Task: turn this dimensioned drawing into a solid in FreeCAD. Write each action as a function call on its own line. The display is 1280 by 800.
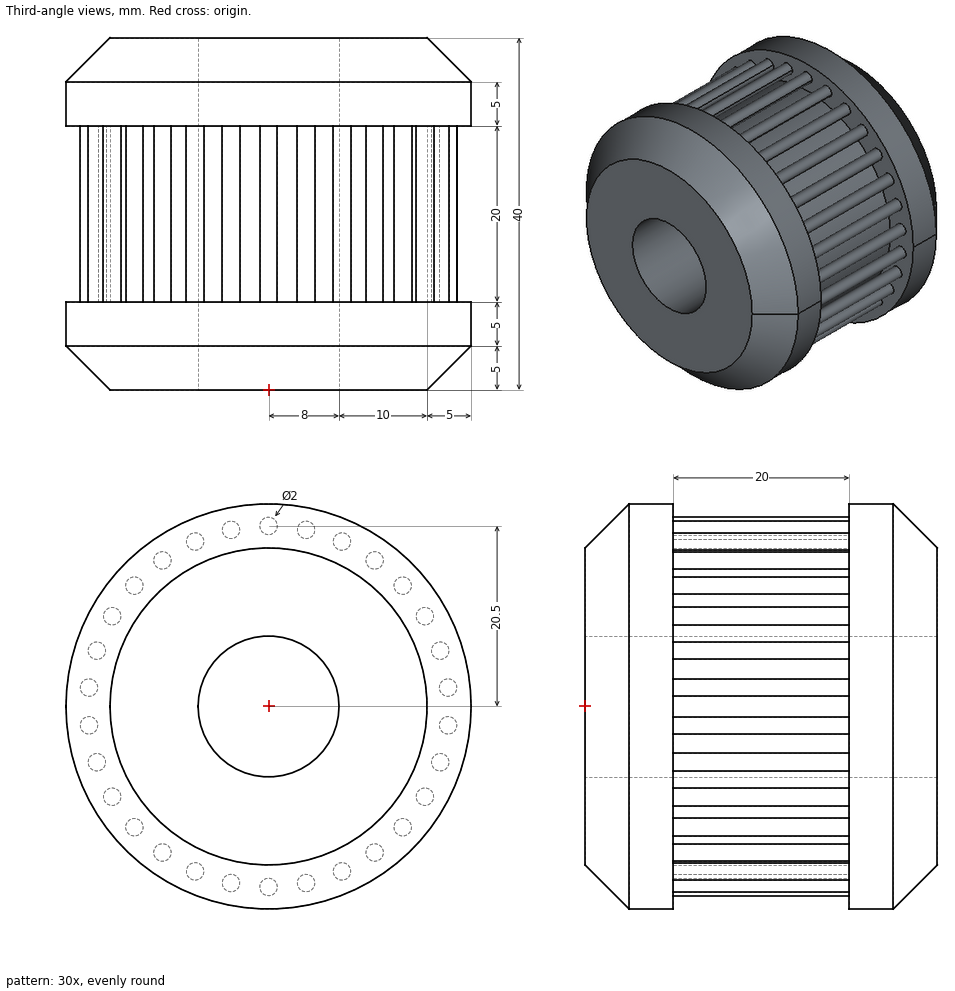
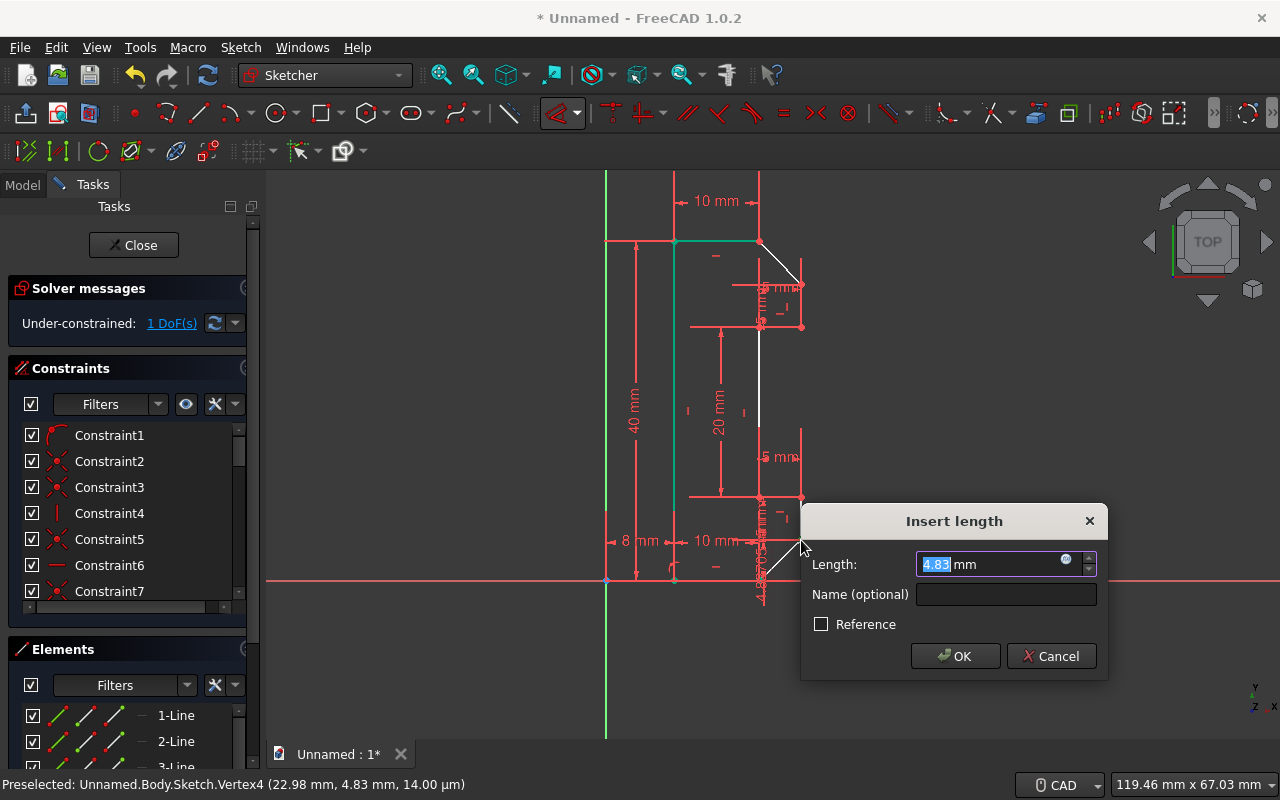
text(5)
key(Return)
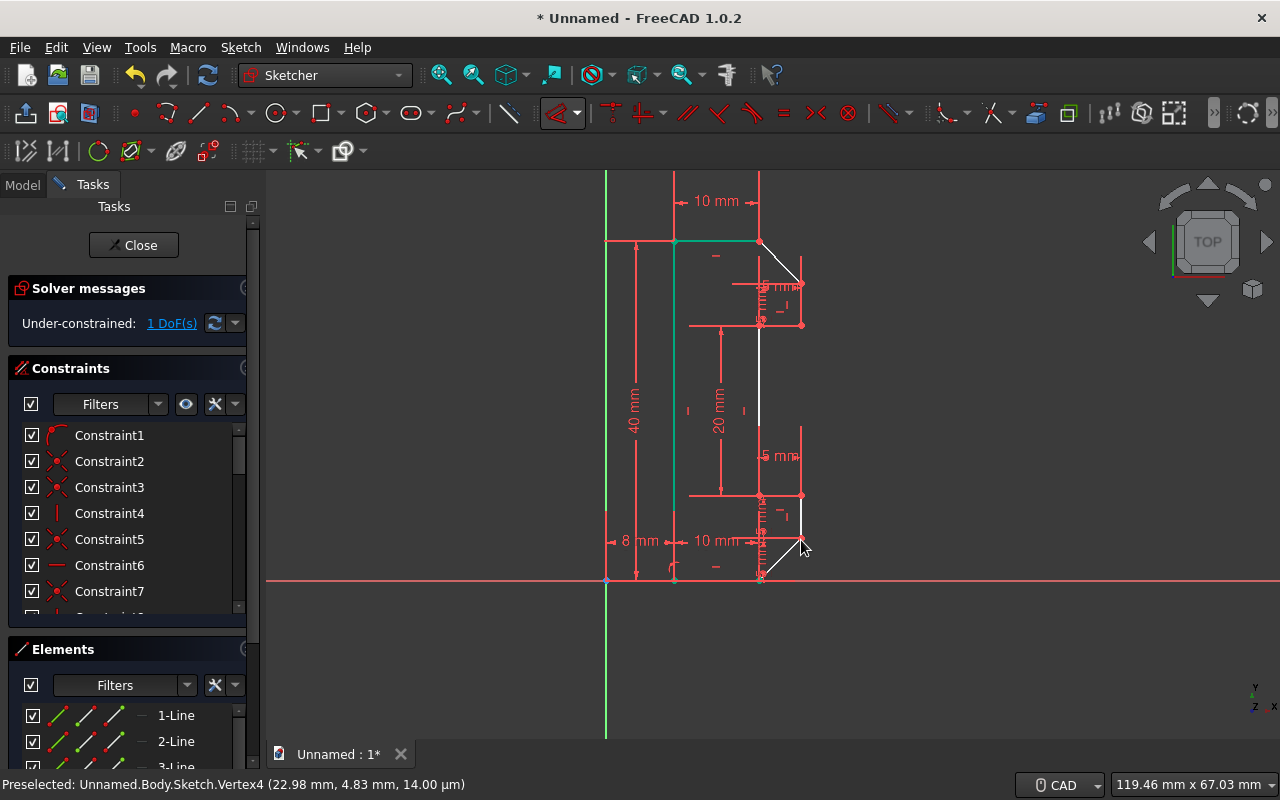
click(772, 568)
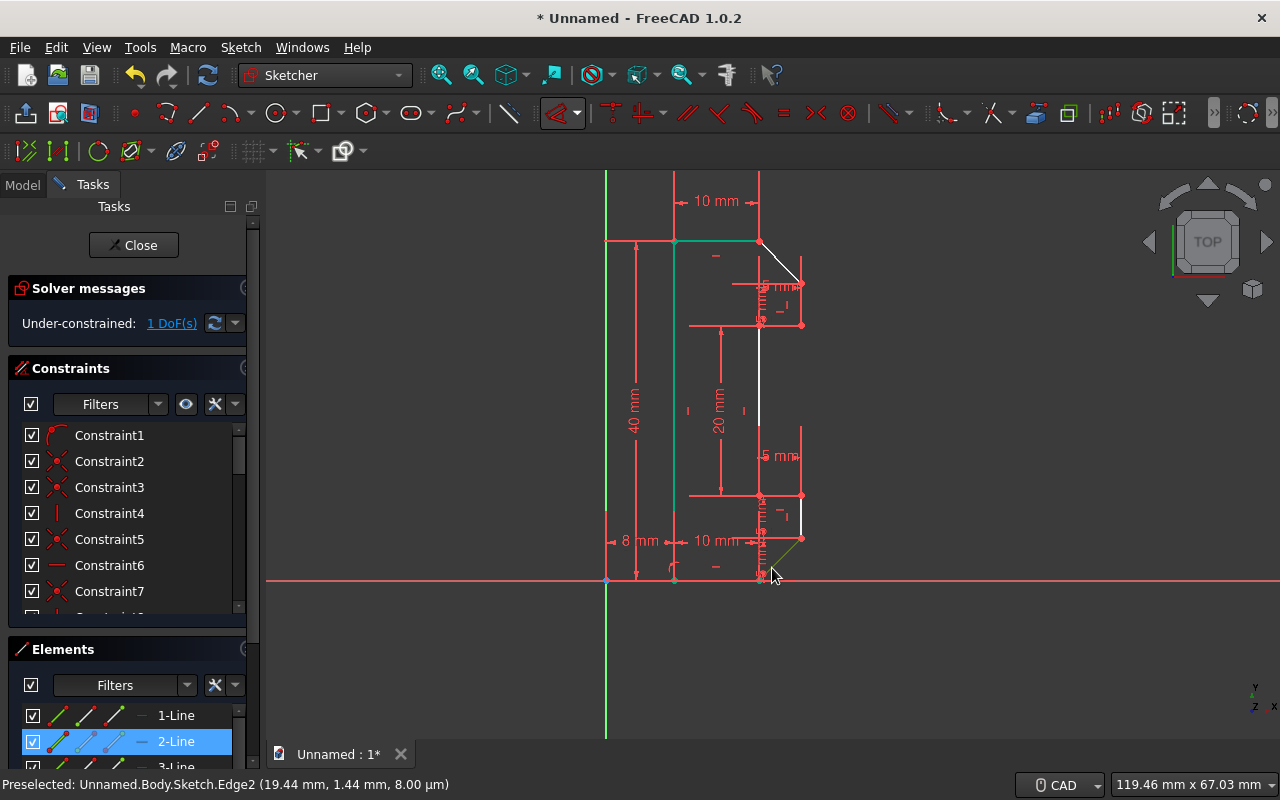
key(l)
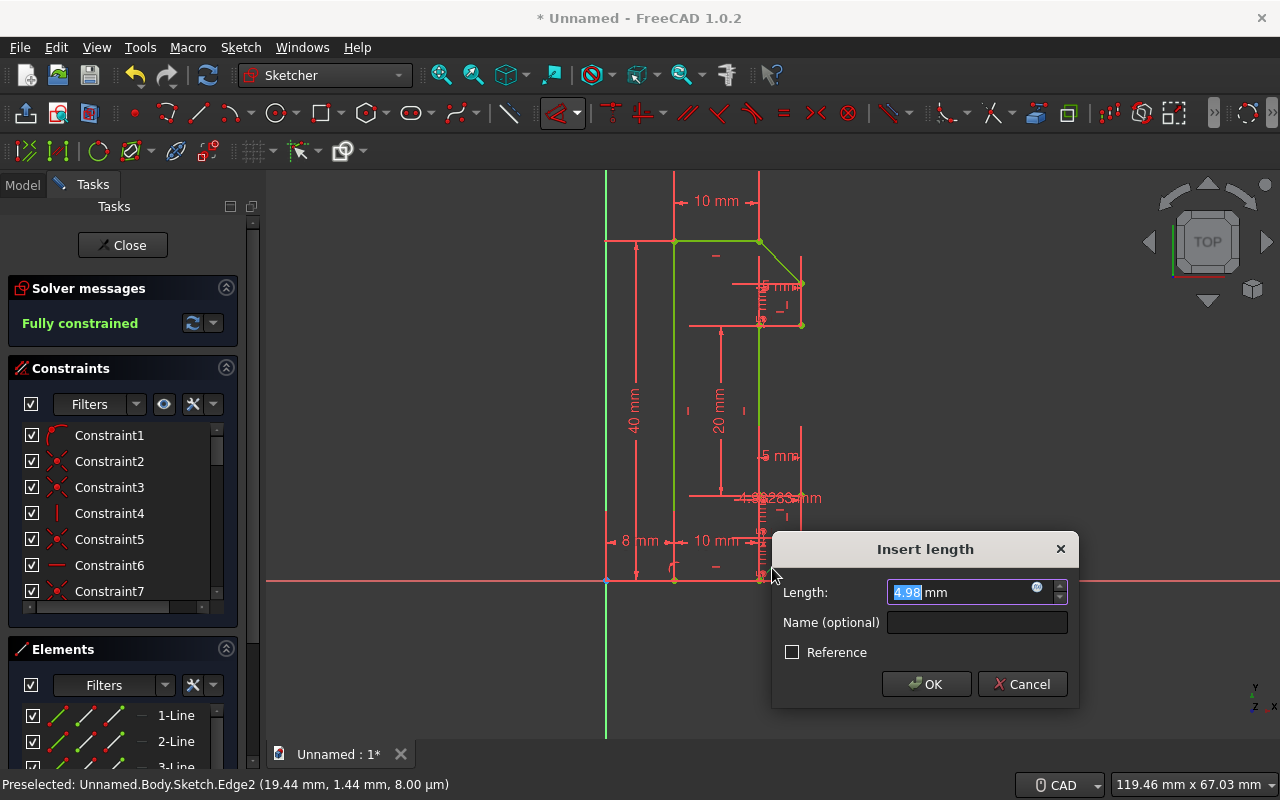
text(5)
key(Return)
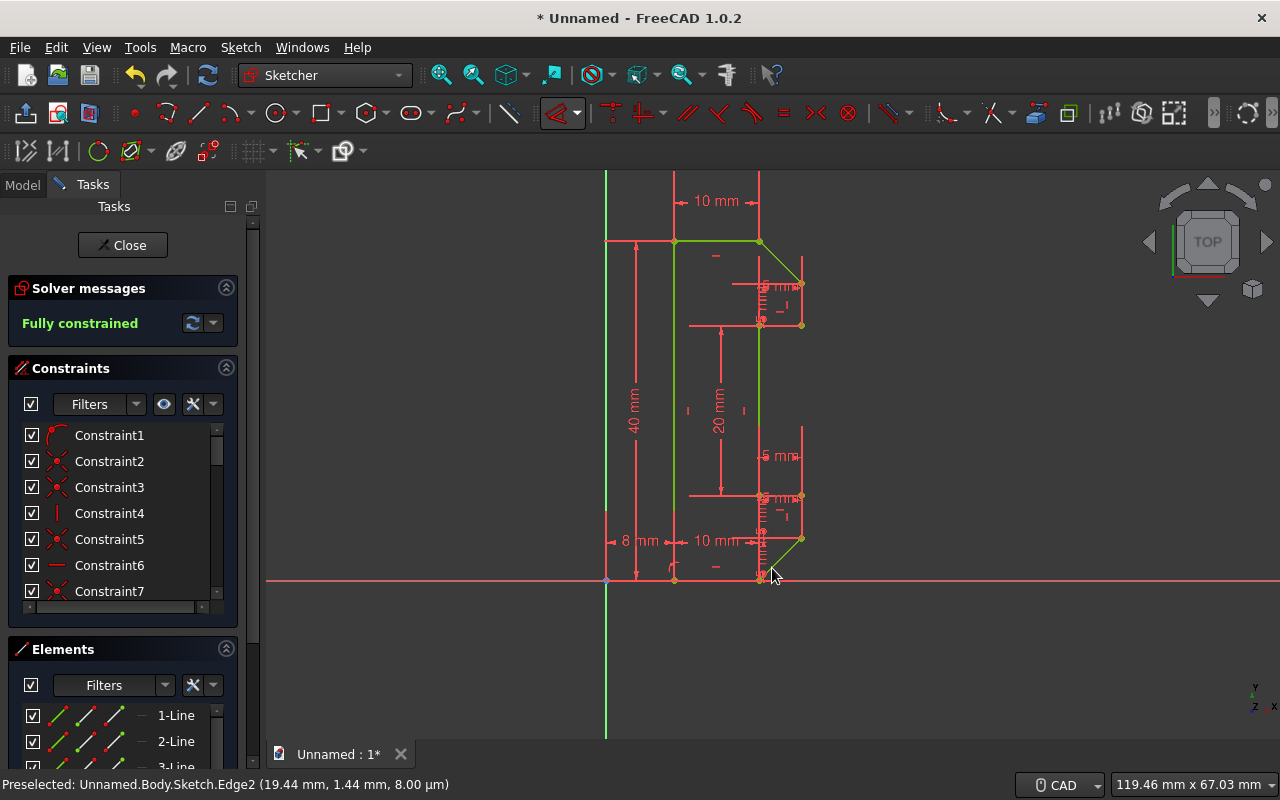
click(123, 245)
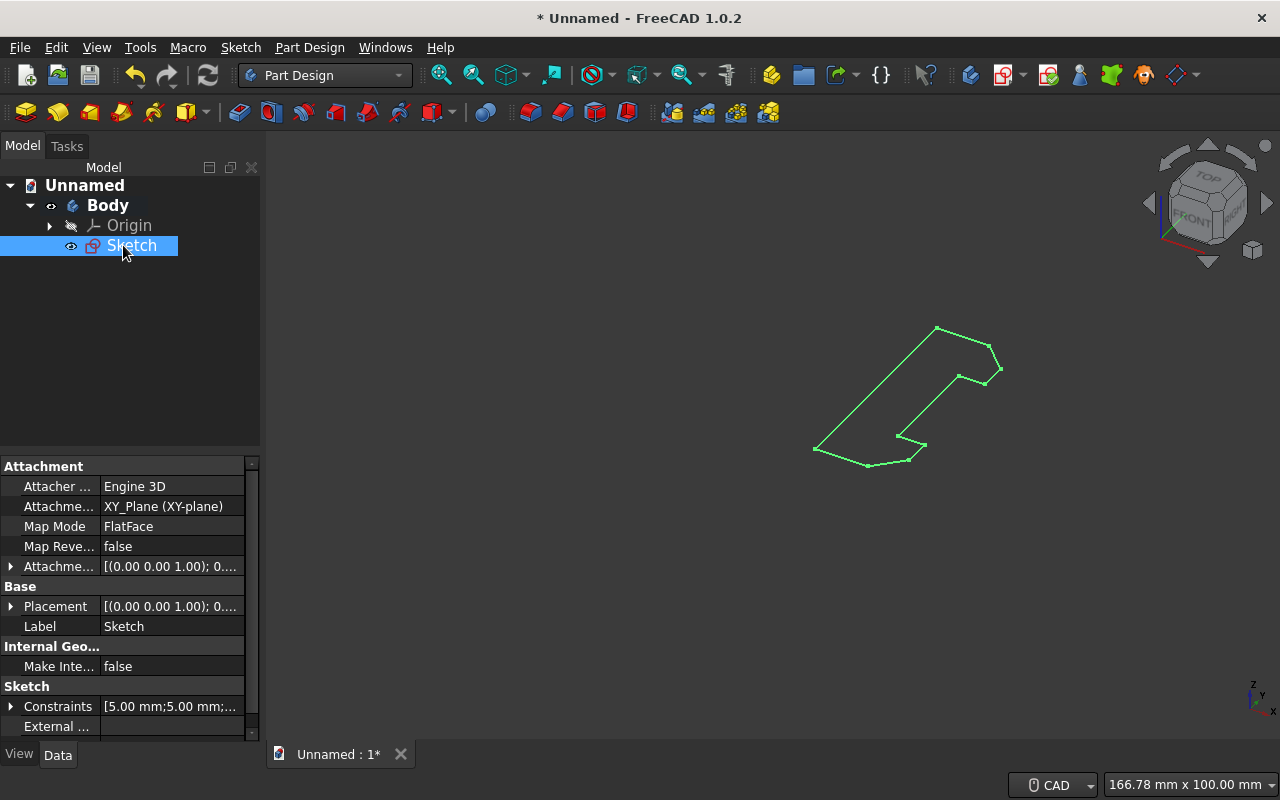
click(58, 112)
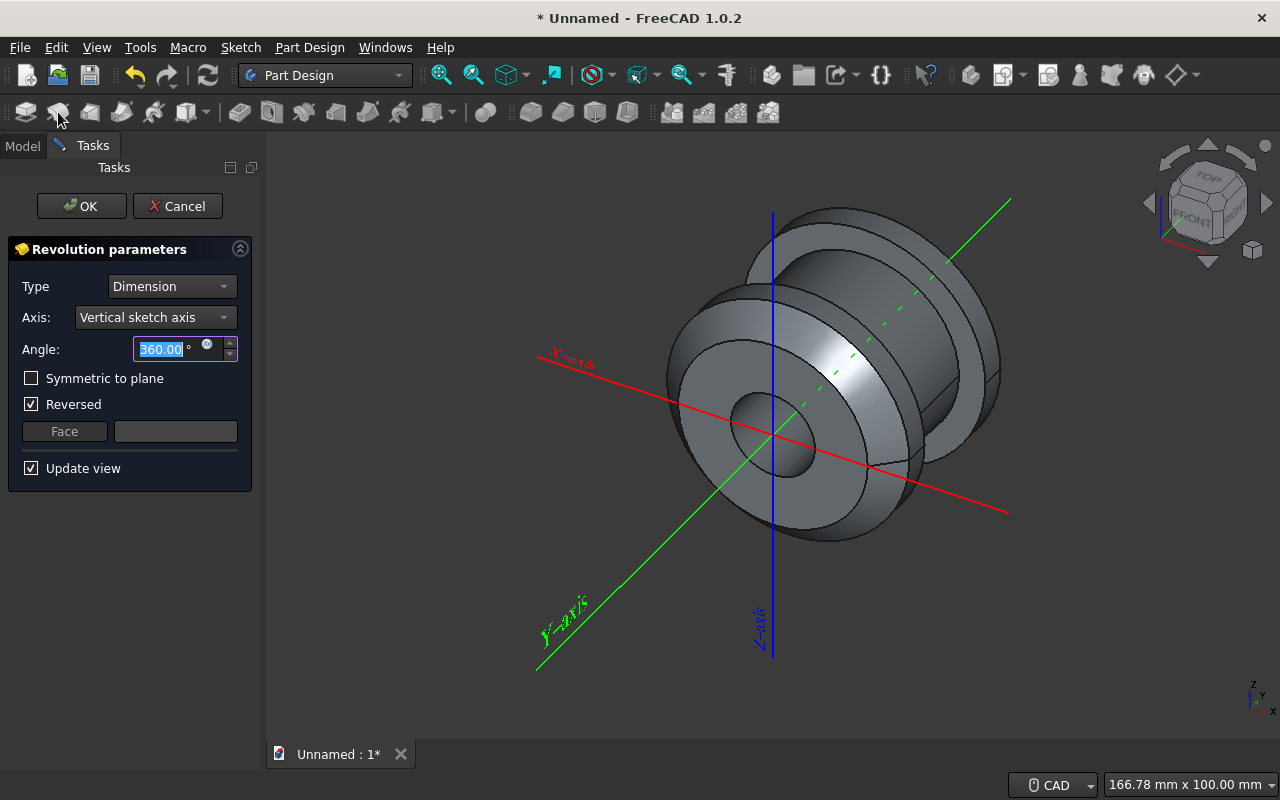
click(82, 206)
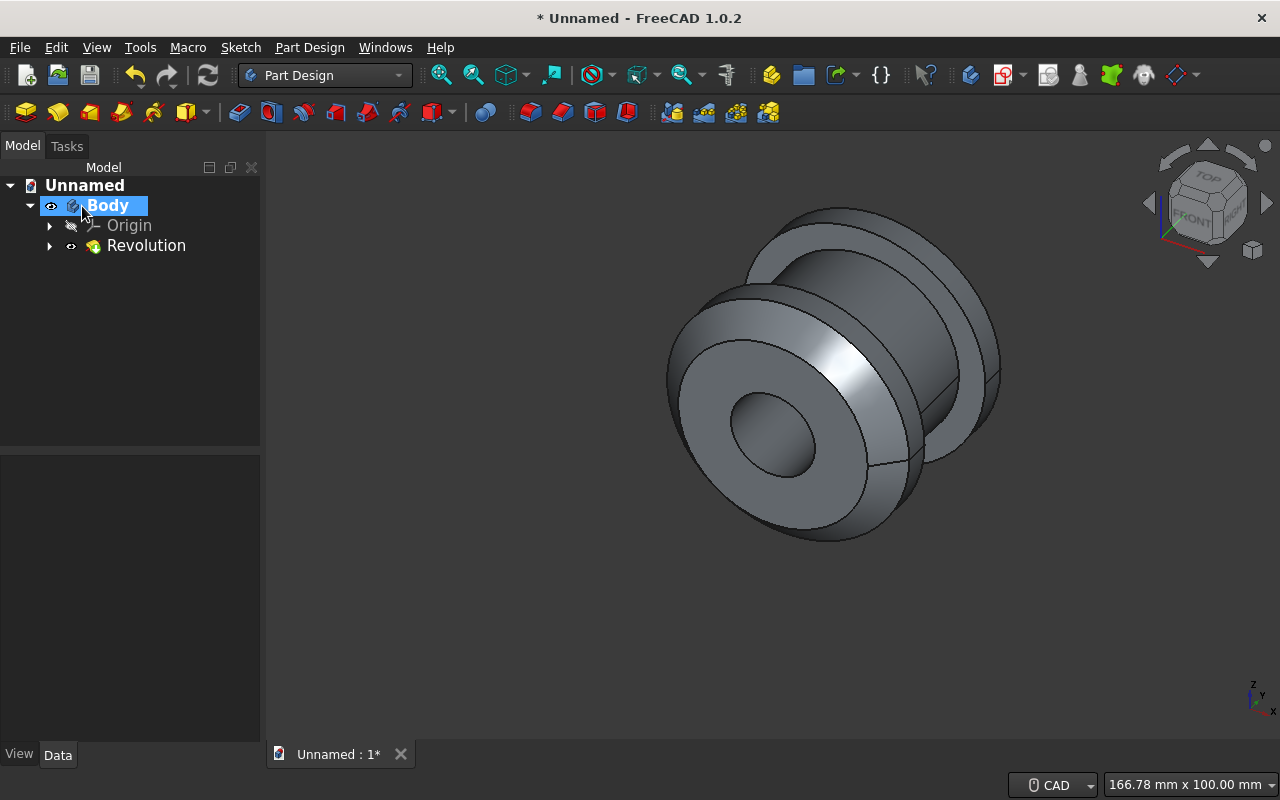
click(50, 226)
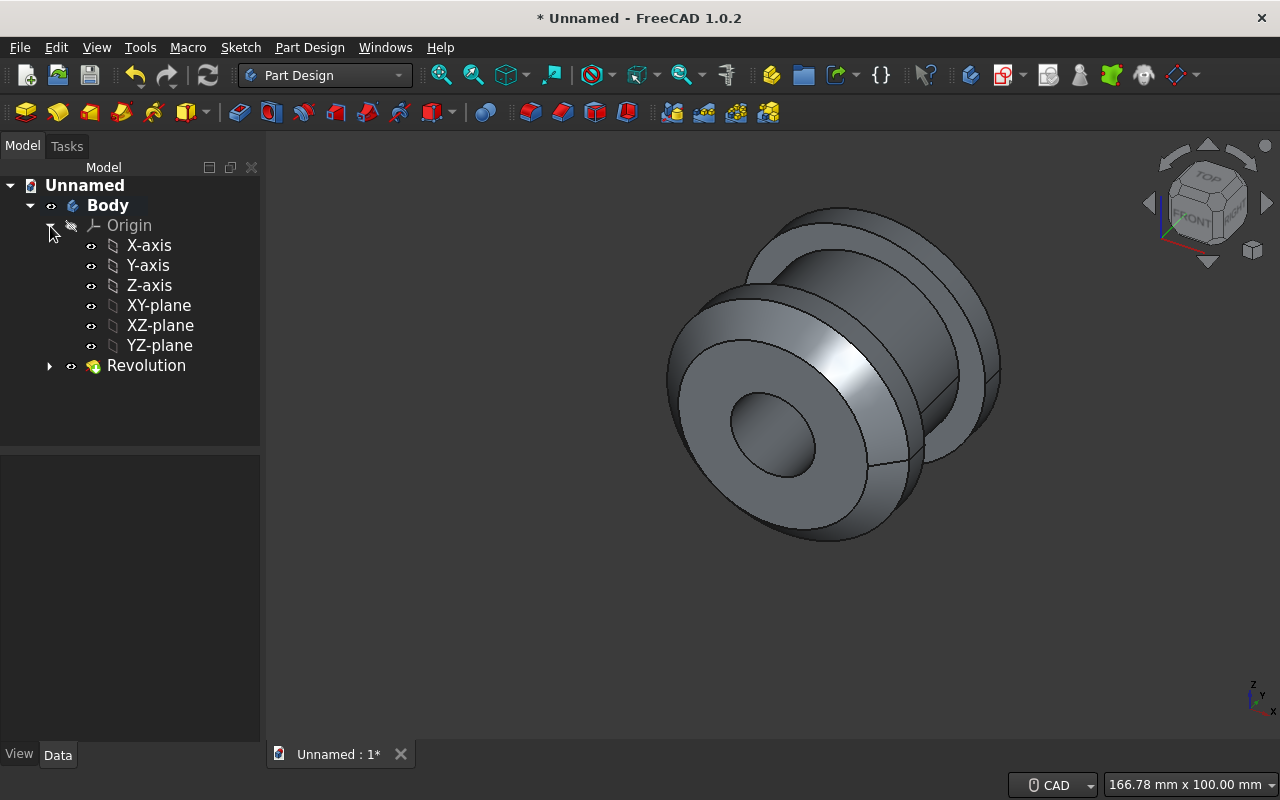
click(136, 326)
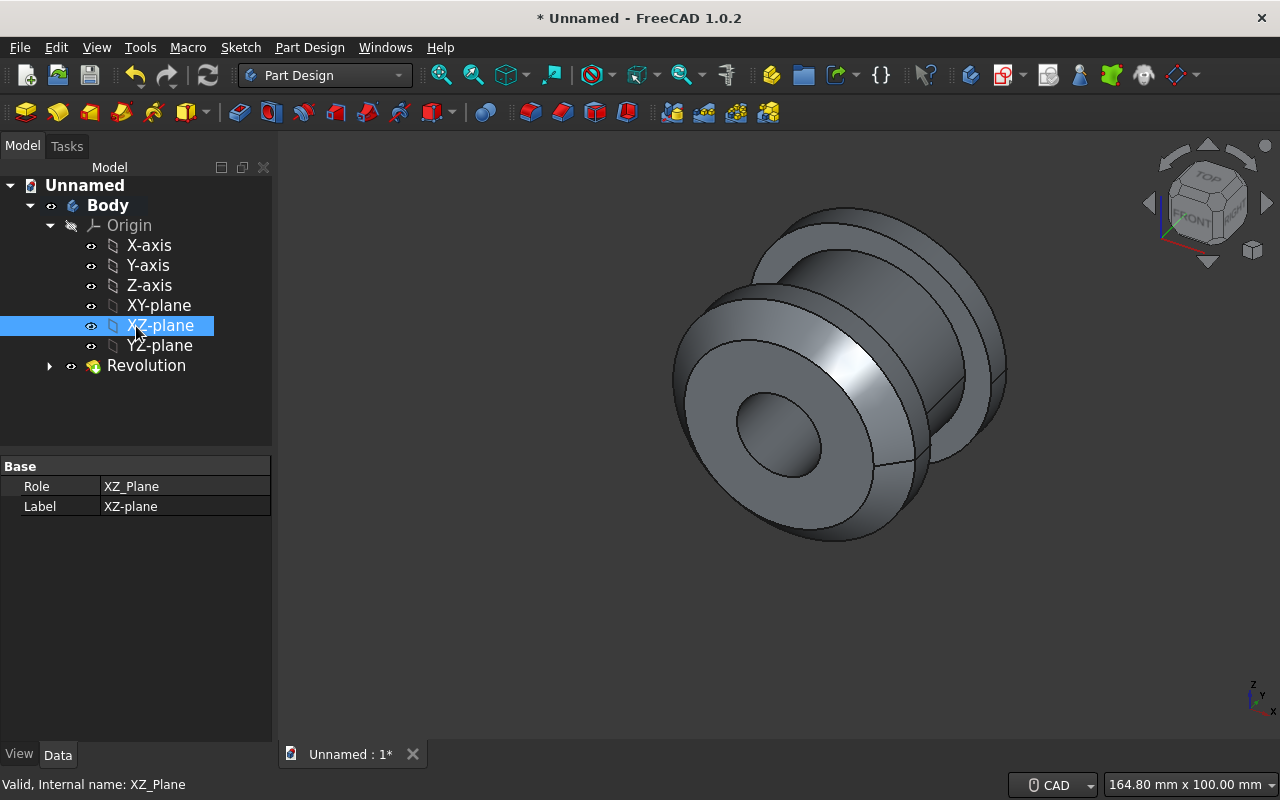
click(1176, 76)